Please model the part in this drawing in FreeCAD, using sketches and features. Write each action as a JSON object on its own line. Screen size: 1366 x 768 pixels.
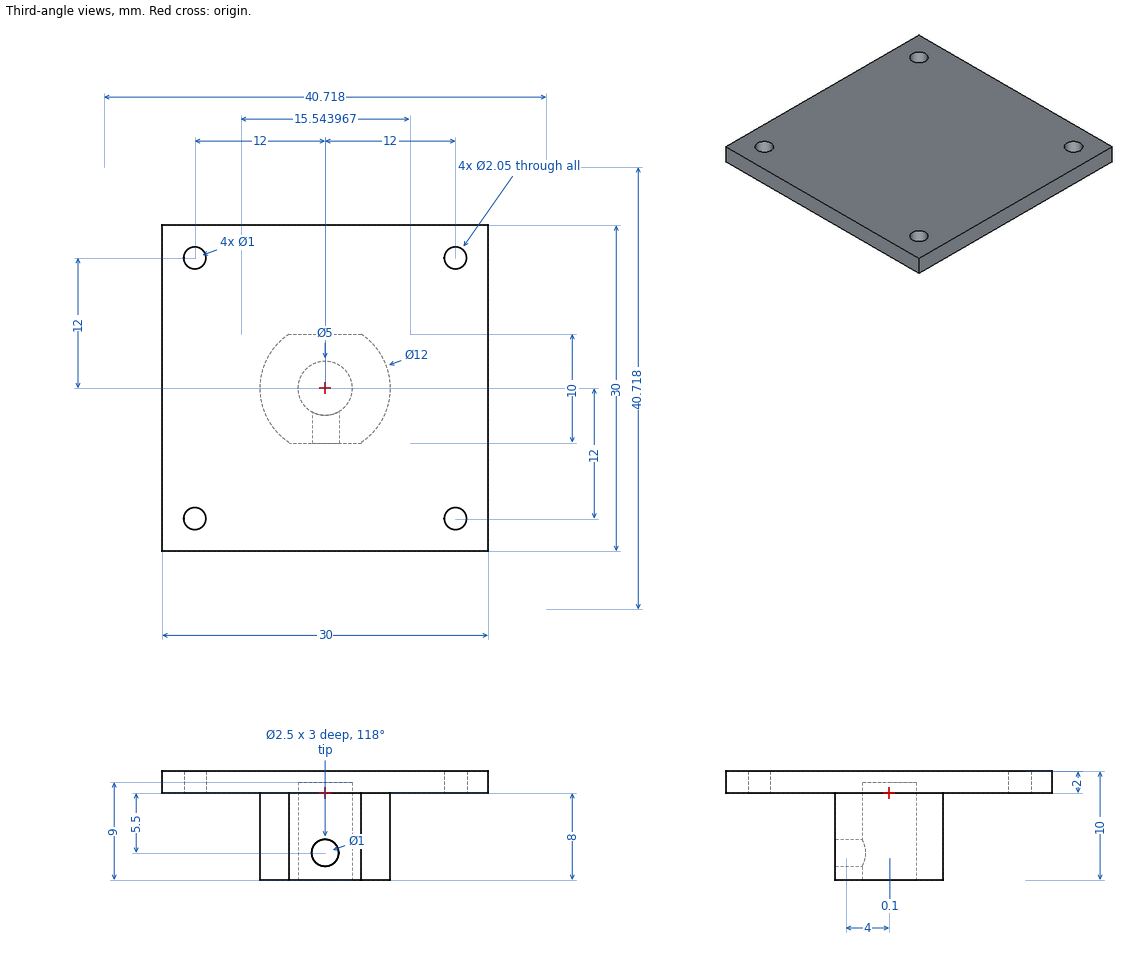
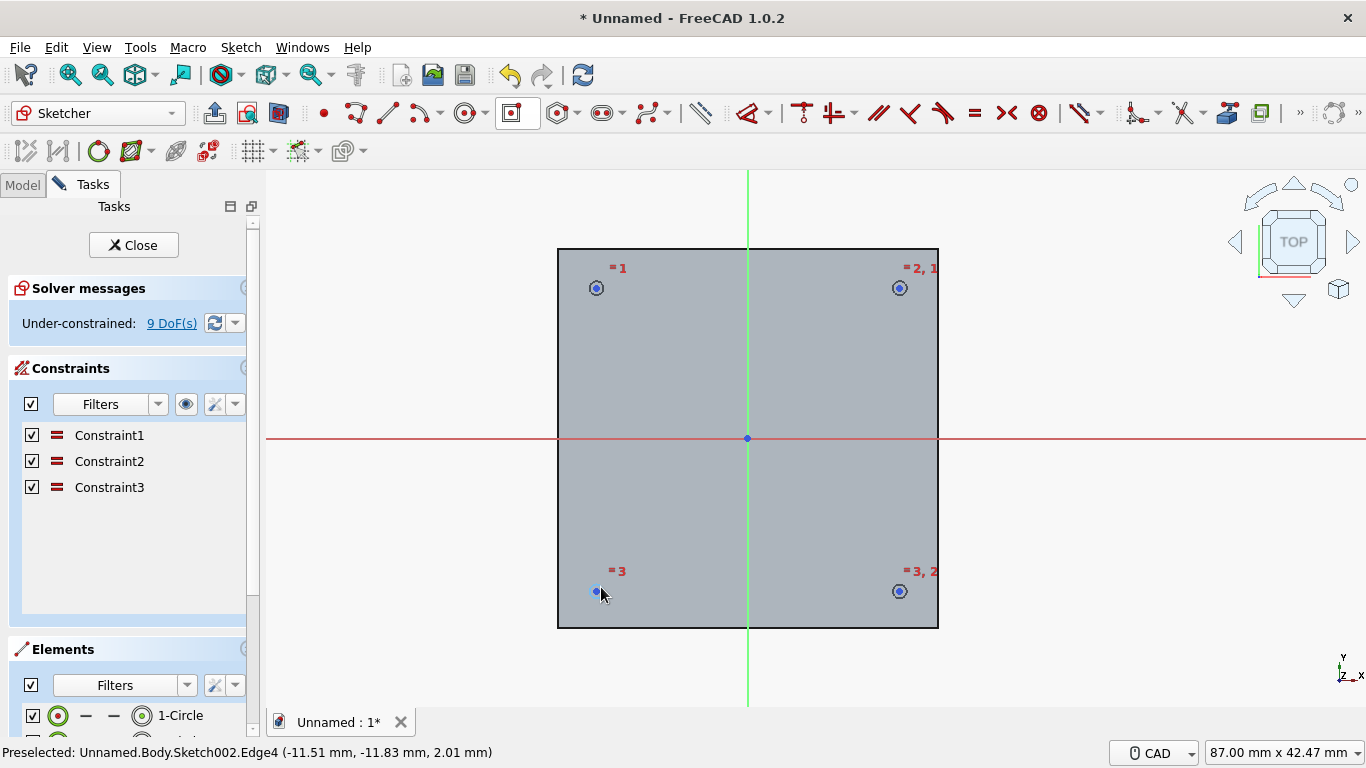
{"action": "left_click", "coordinate": [597, 288]}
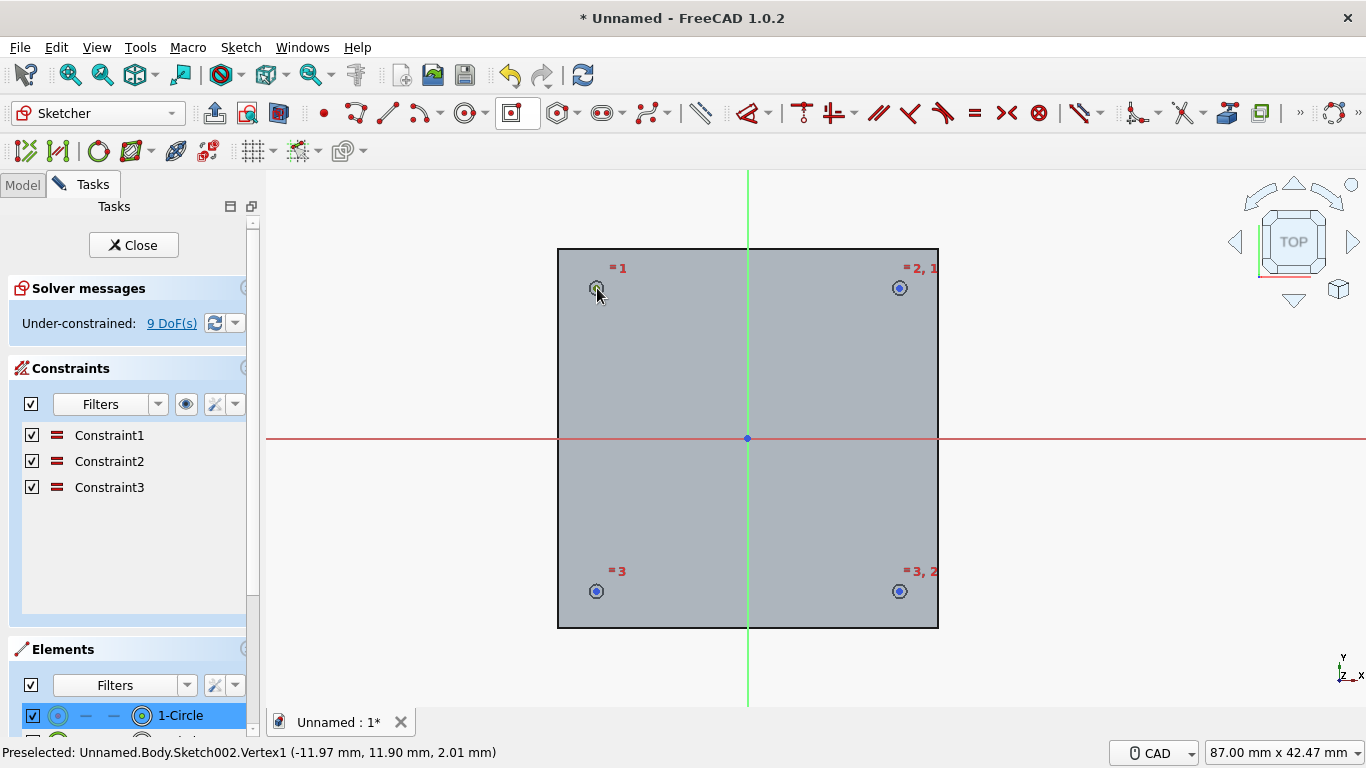
{"action": "left_click", "coordinate": [900, 288]}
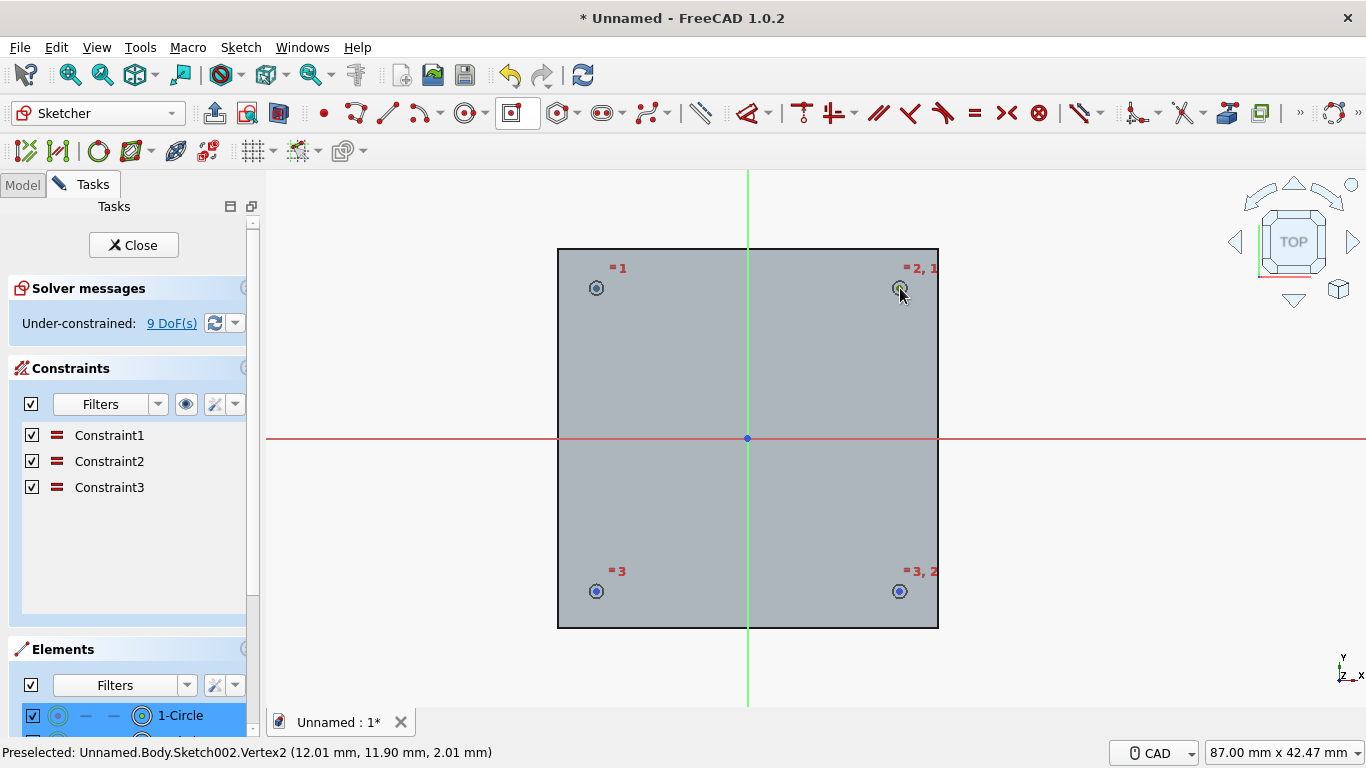
{"action": "key", "text": "h"}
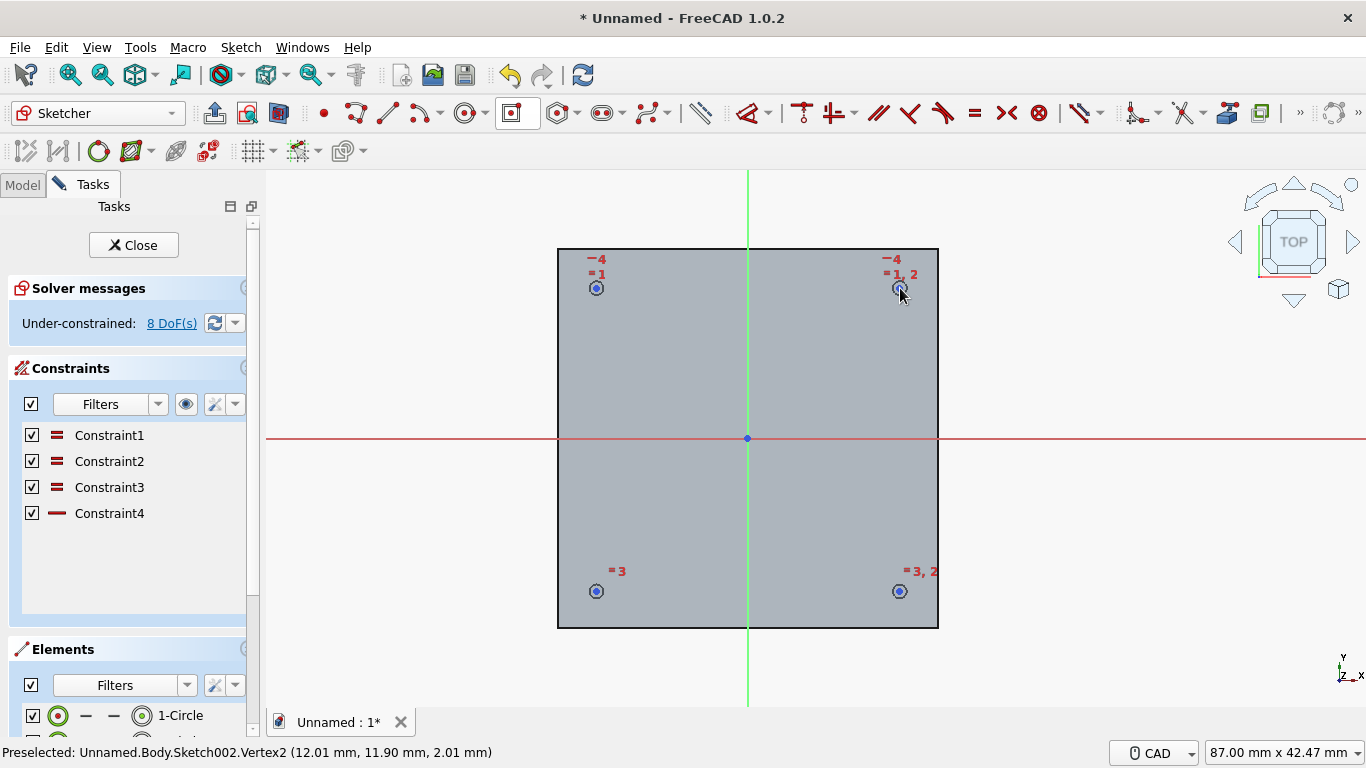
{"action": "left_click", "coordinate": [900, 288]}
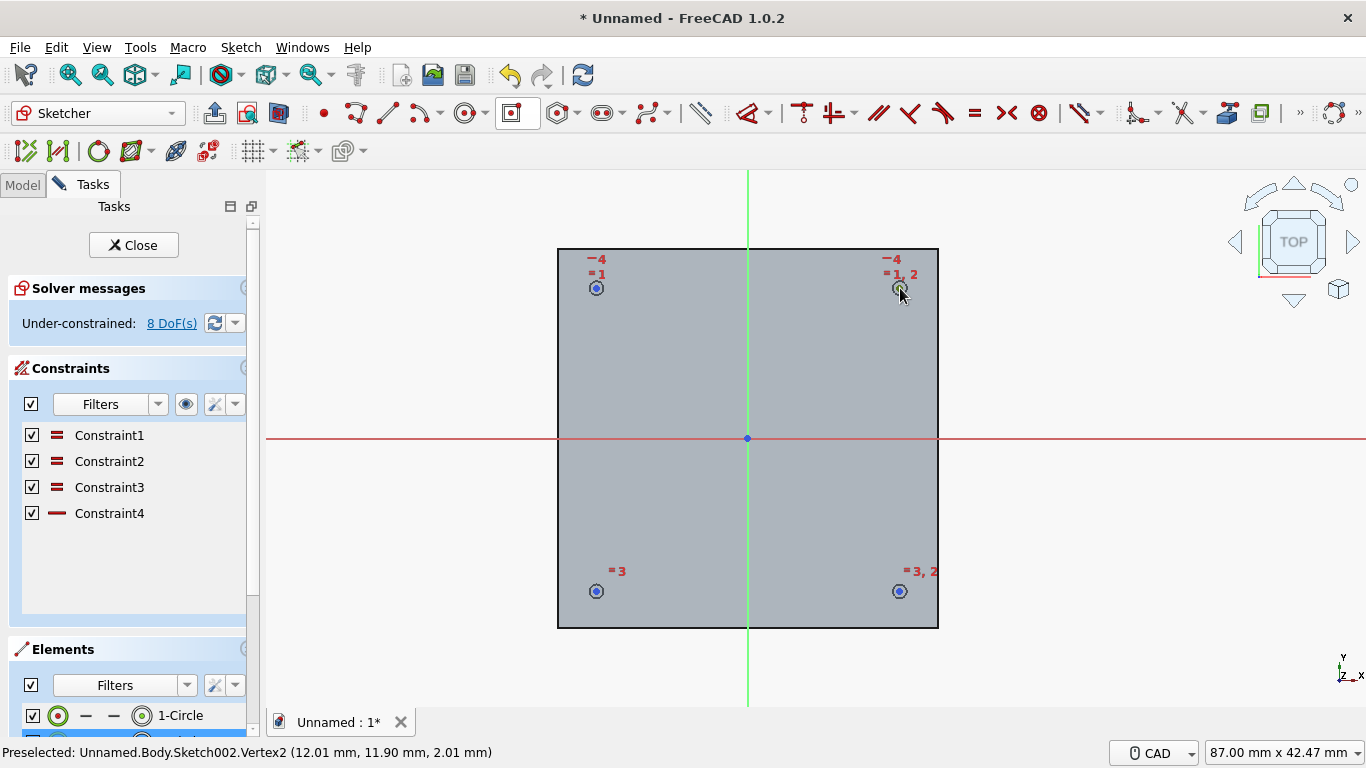
{"action": "left_click", "coordinate": [900, 591]}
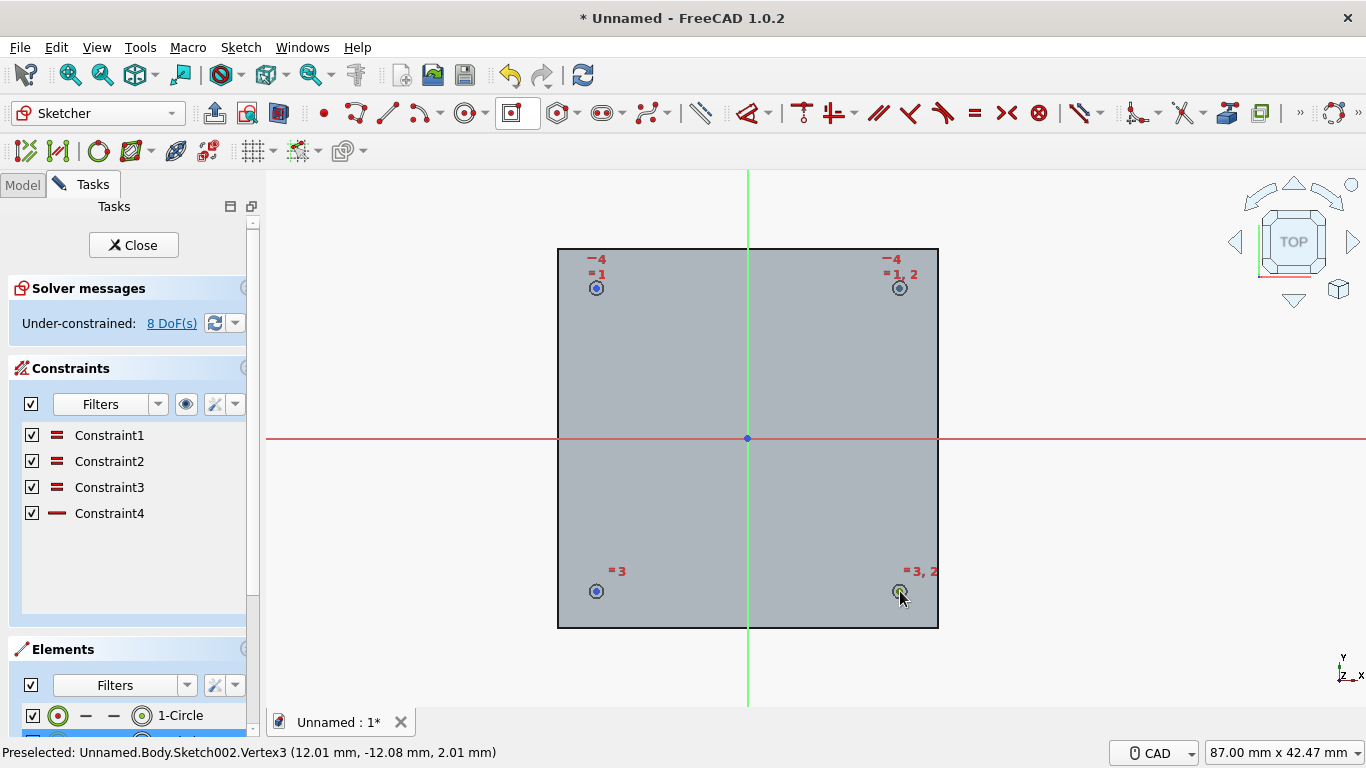
{"action": "key", "text": "v"}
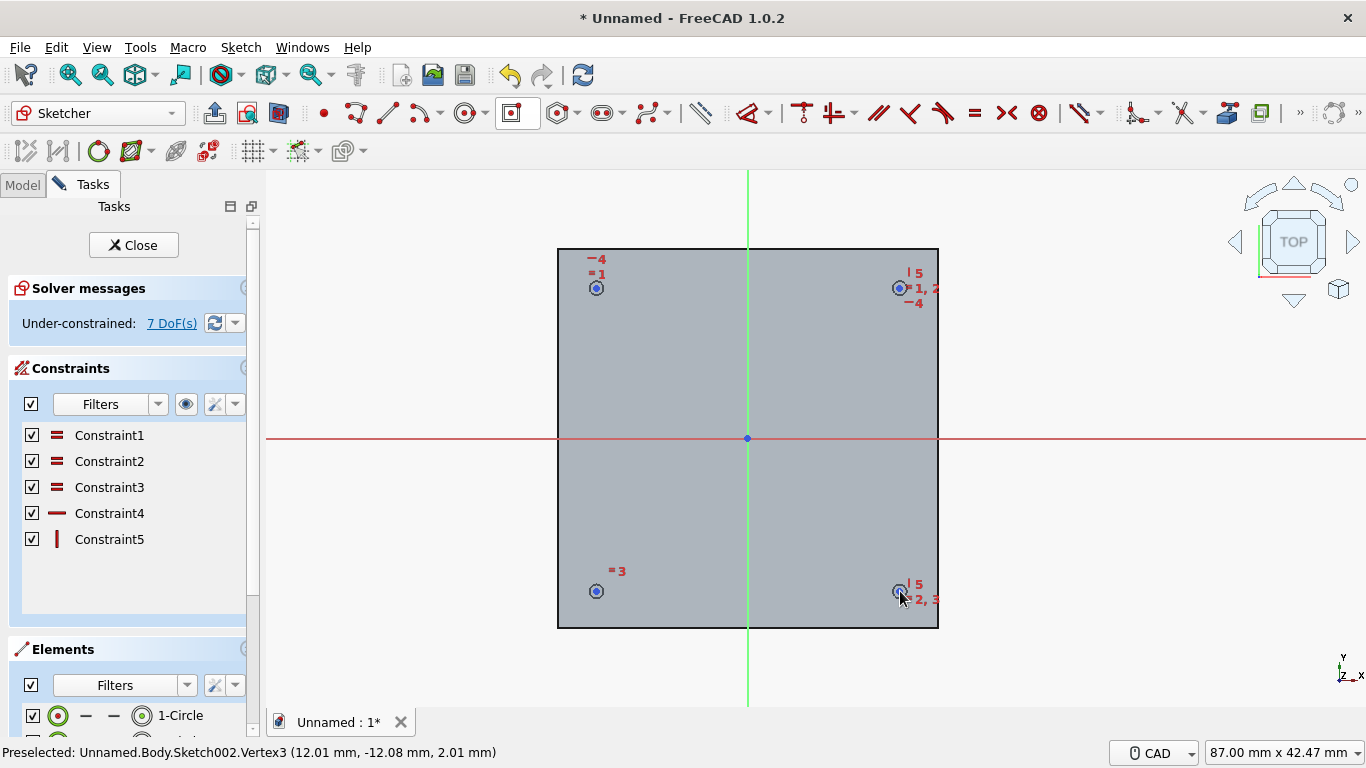
{"action": "left_click", "coordinate": [597, 288]}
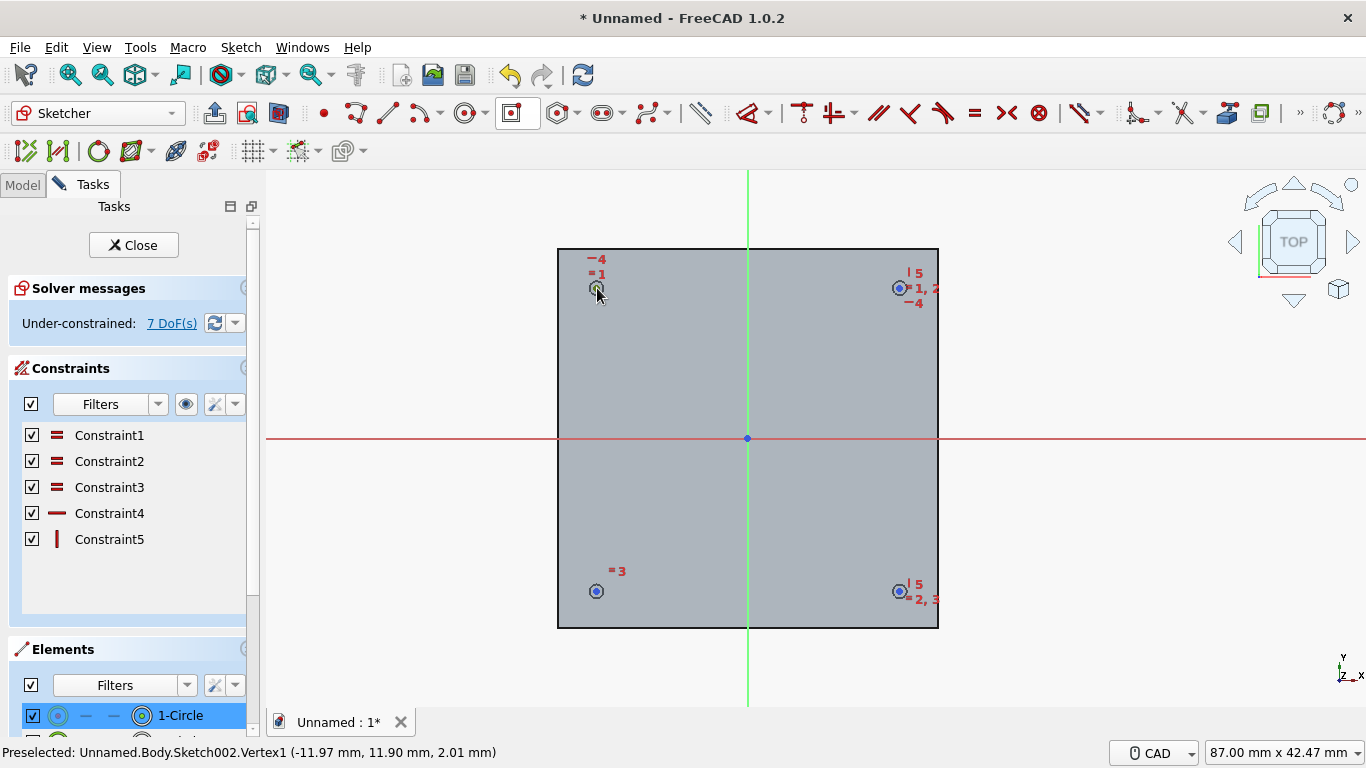
{"action": "left_click", "coordinate": [597, 591]}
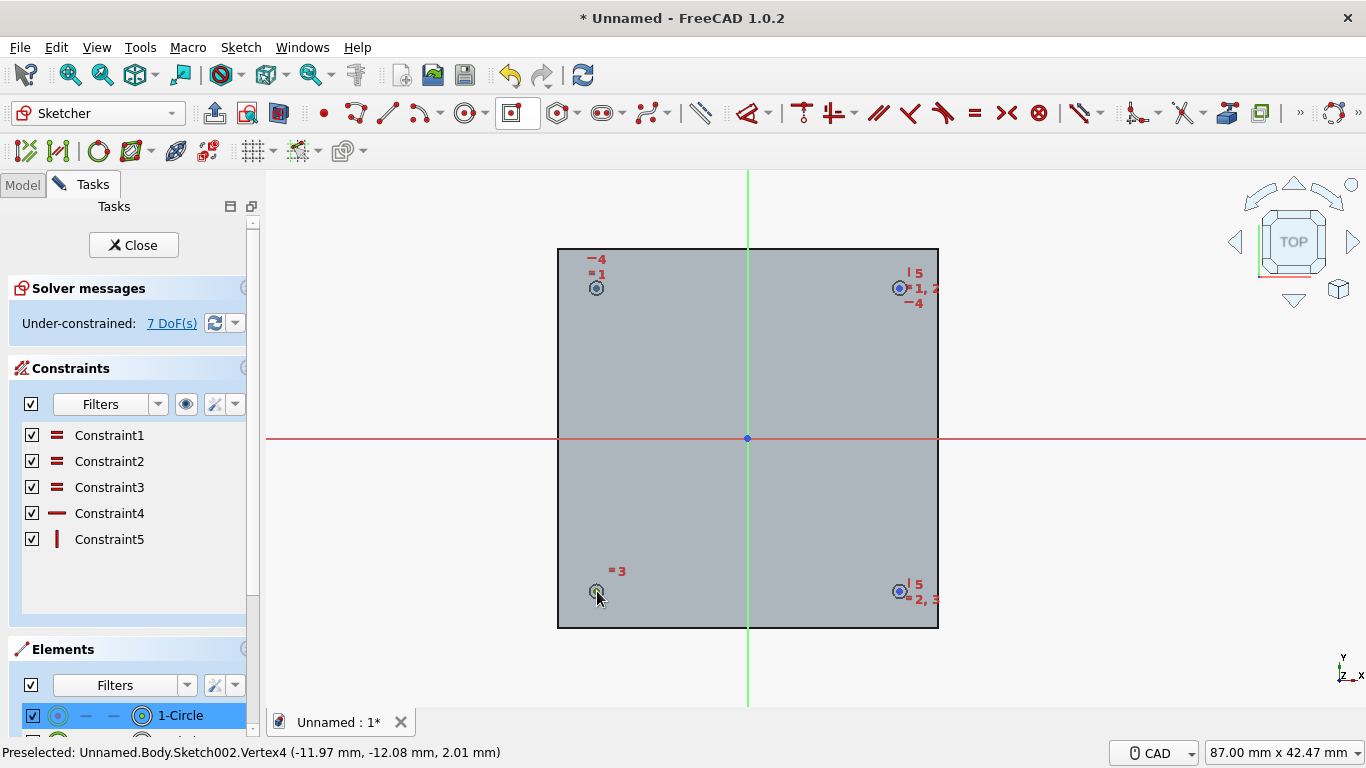
{"action": "key", "text": "v"}